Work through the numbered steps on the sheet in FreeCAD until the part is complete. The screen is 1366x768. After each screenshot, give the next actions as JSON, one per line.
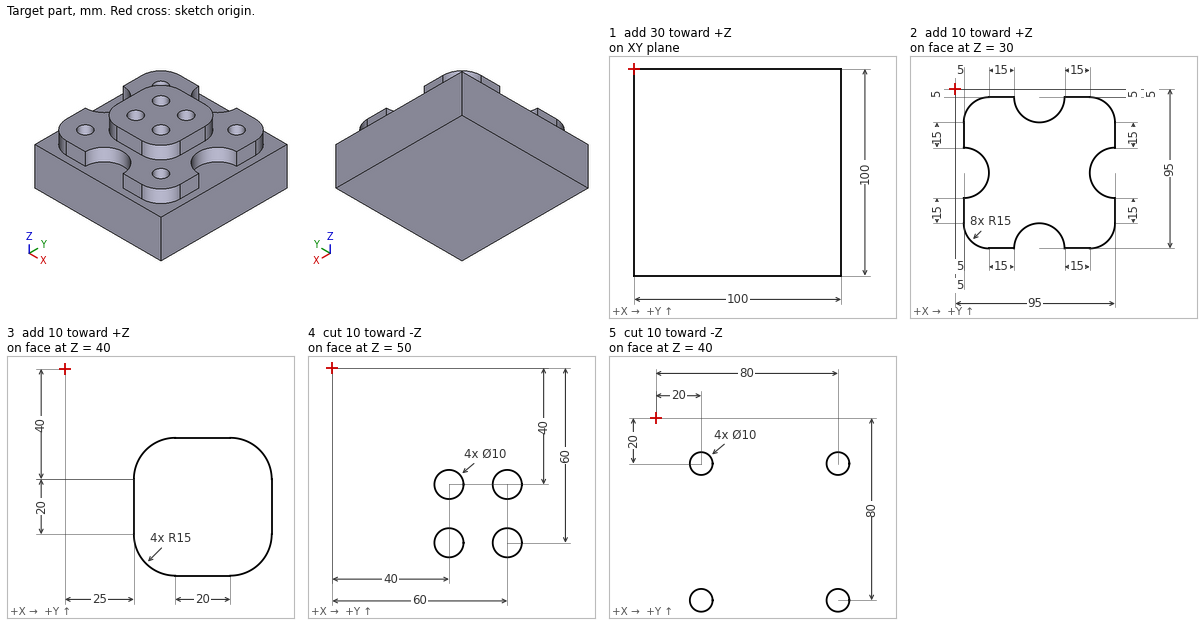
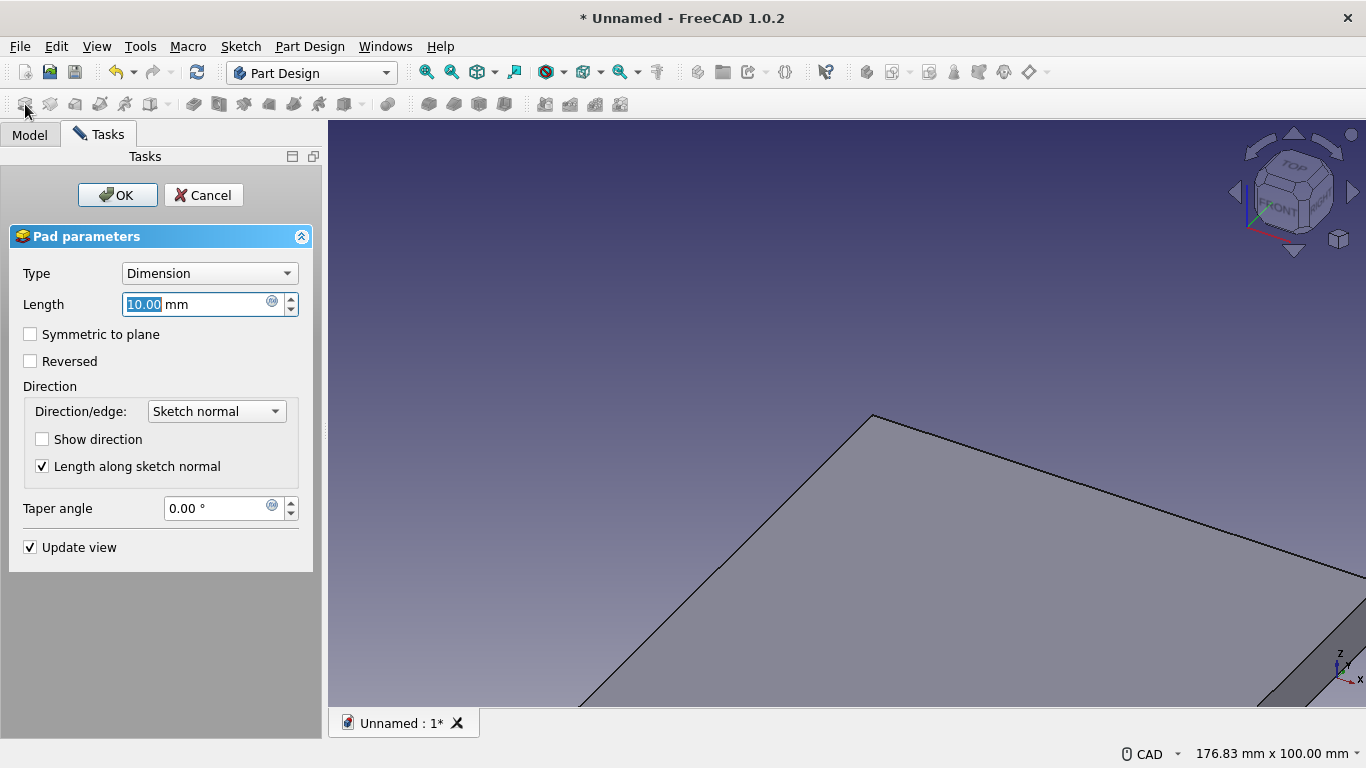
{"action": "type", "text": "30"}
{"action": "key", "text": "Tab"}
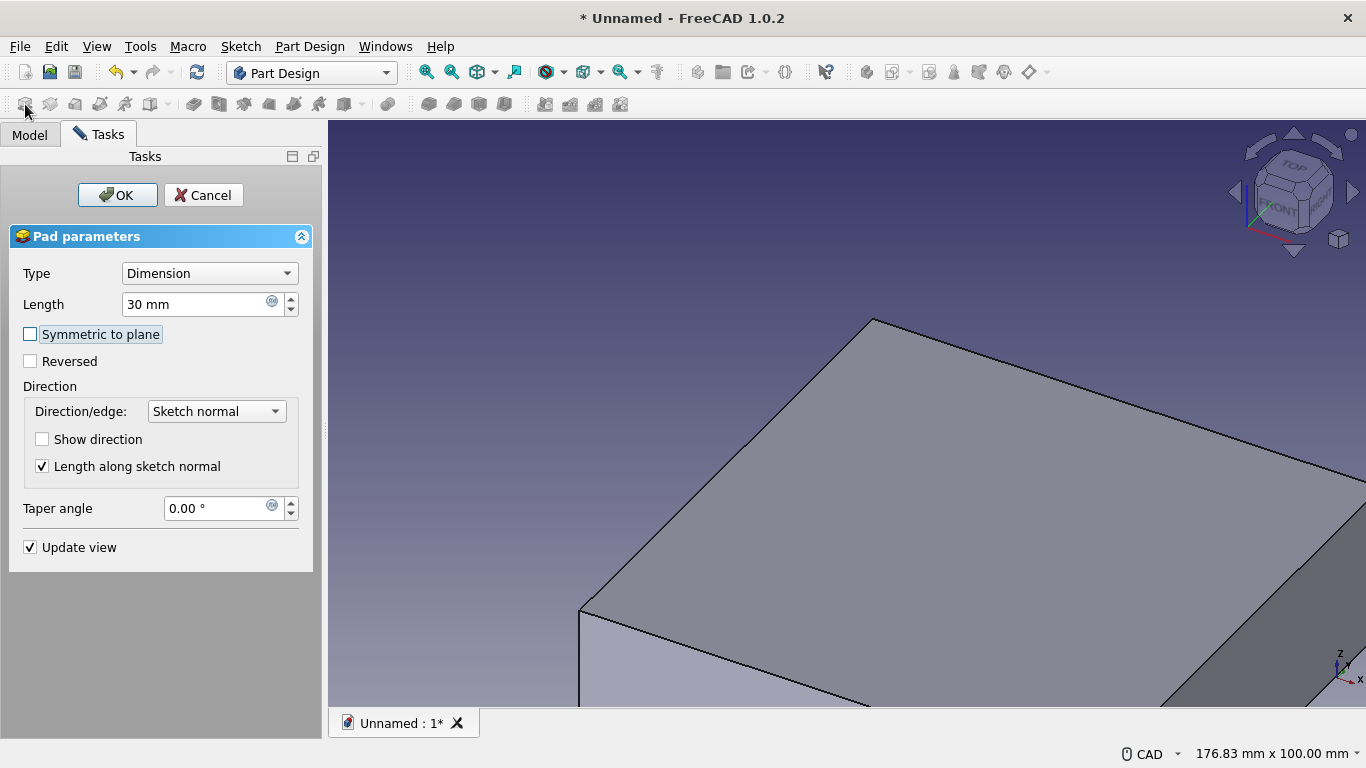
{"action": "left_click", "coordinate": [118, 195]}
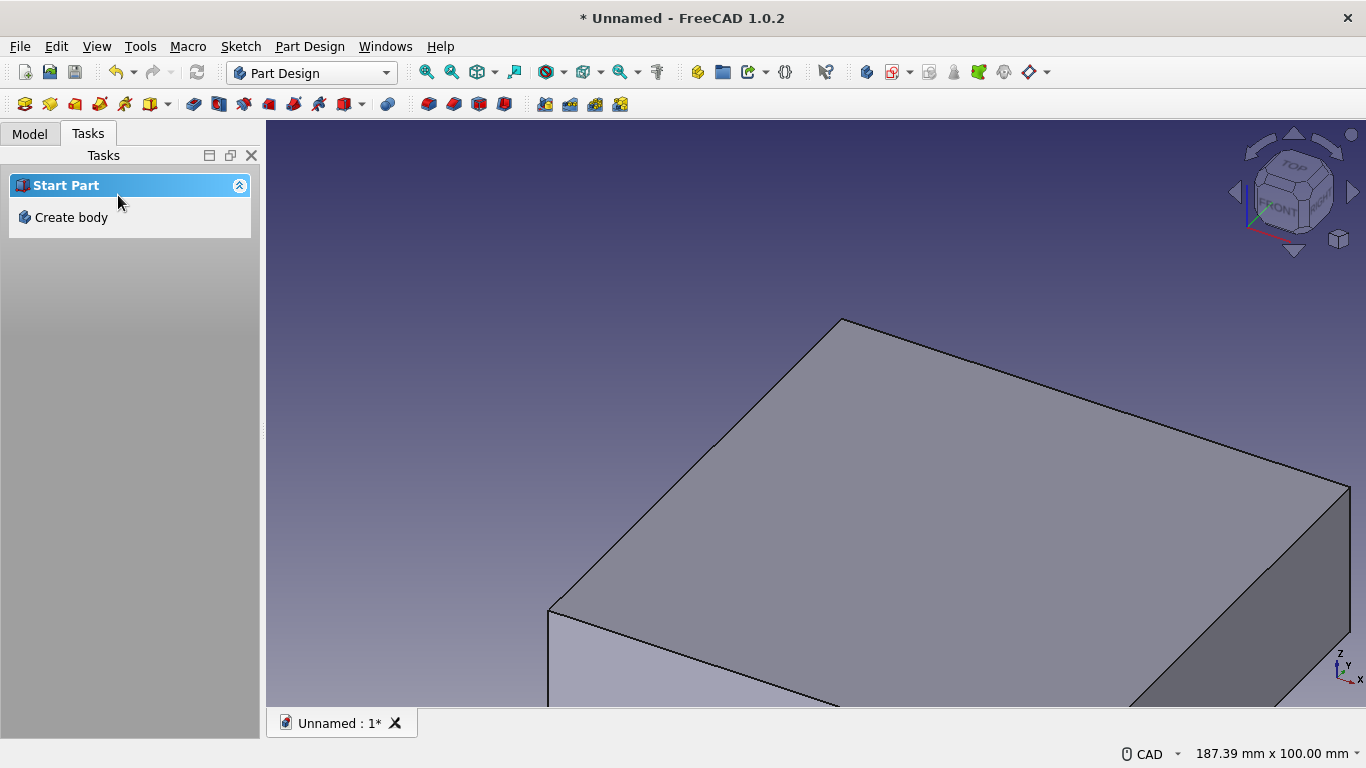
{"action": "left_click", "coordinate": [427, 72]}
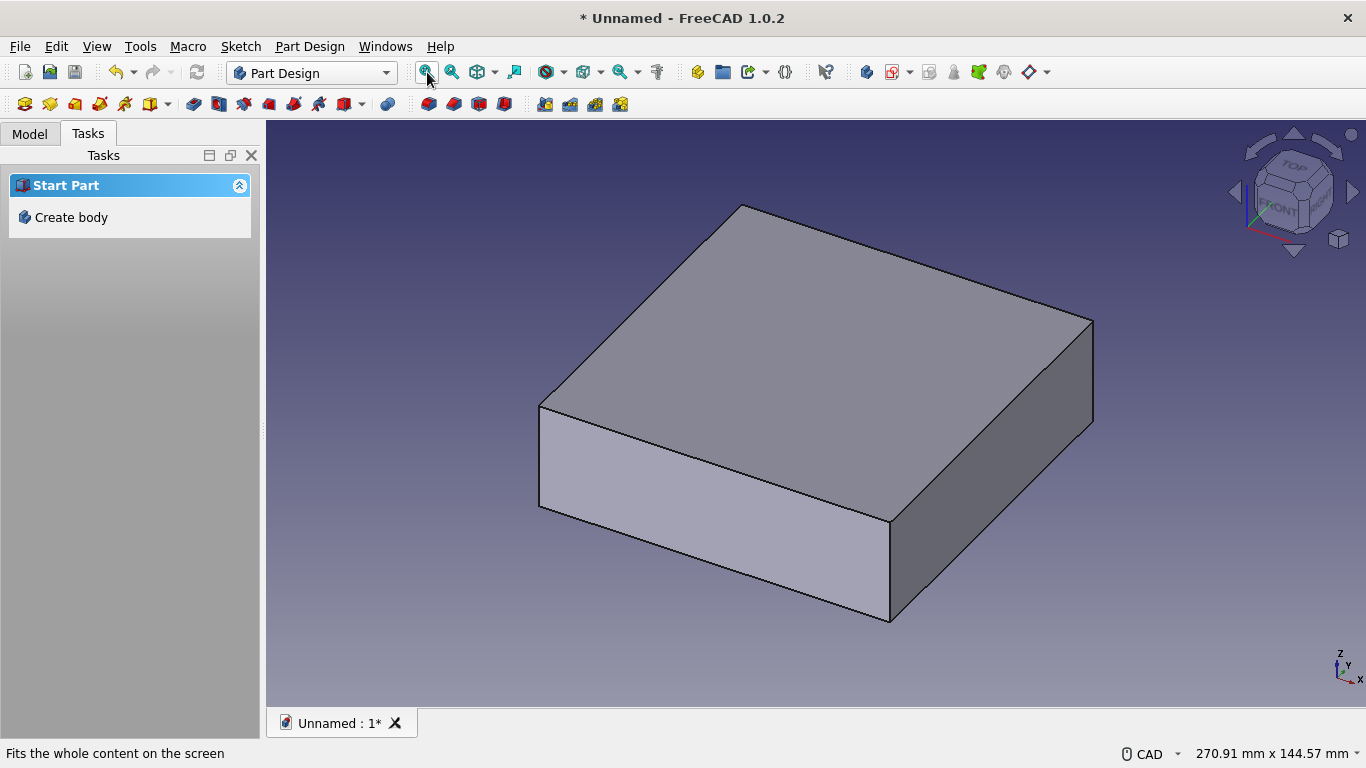
{"action": "left_click", "coordinate": [816, 363]}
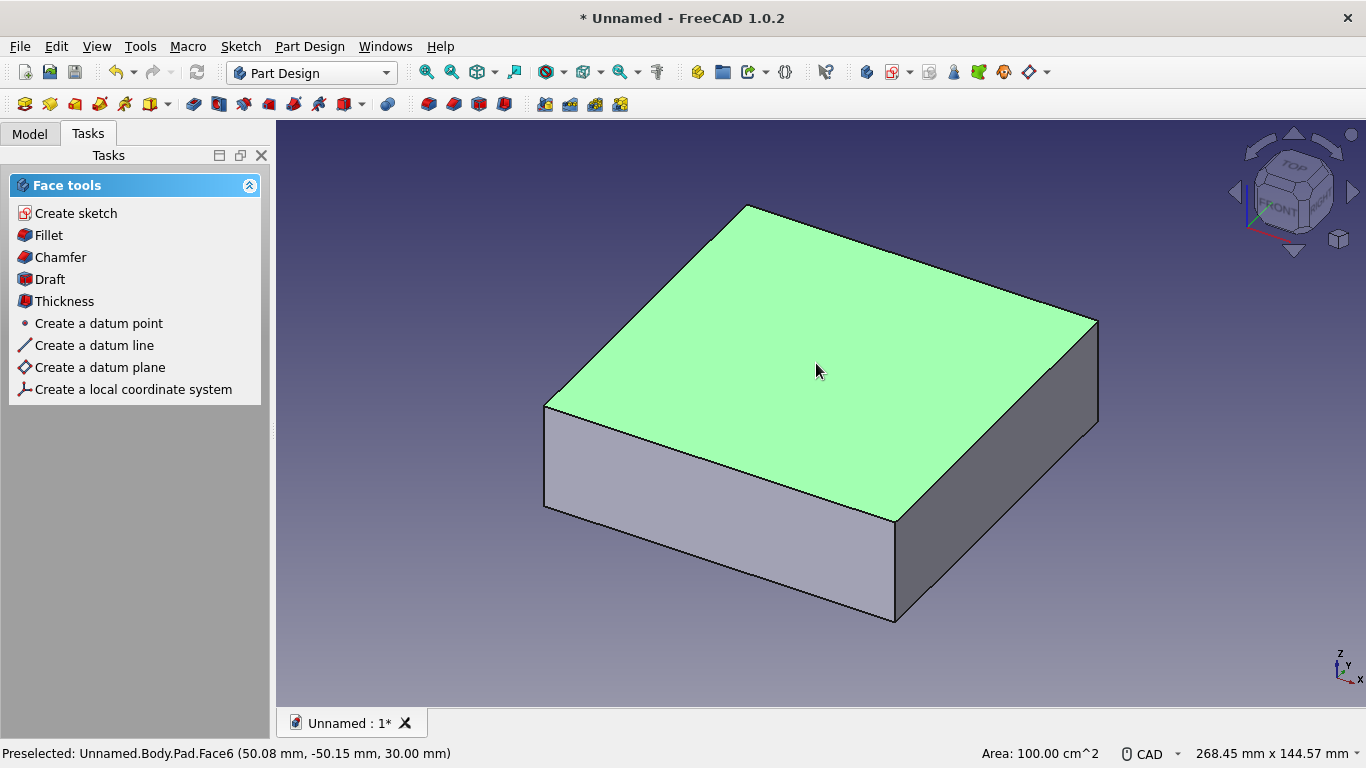
{"action": "left_click", "coordinate": [892, 72]}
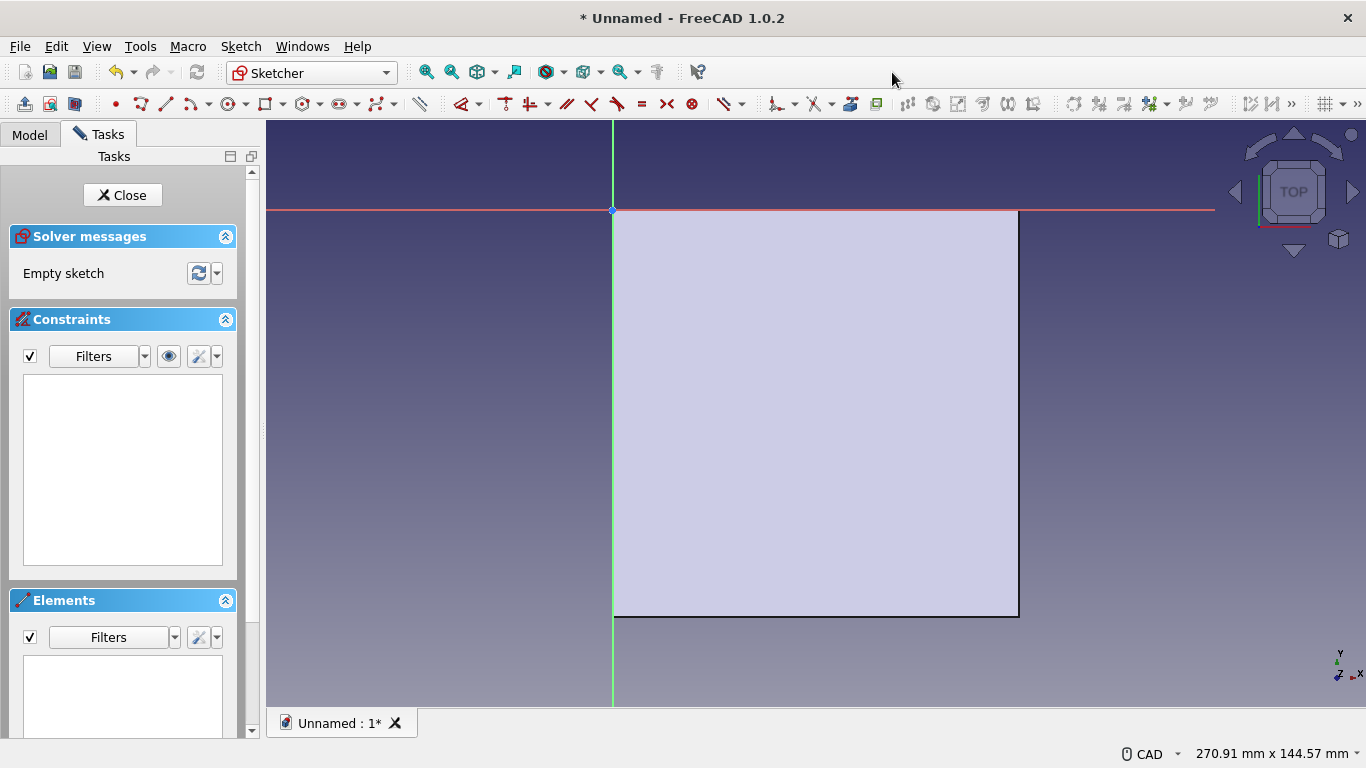
{"action": "left_click", "coordinate": [166, 104]}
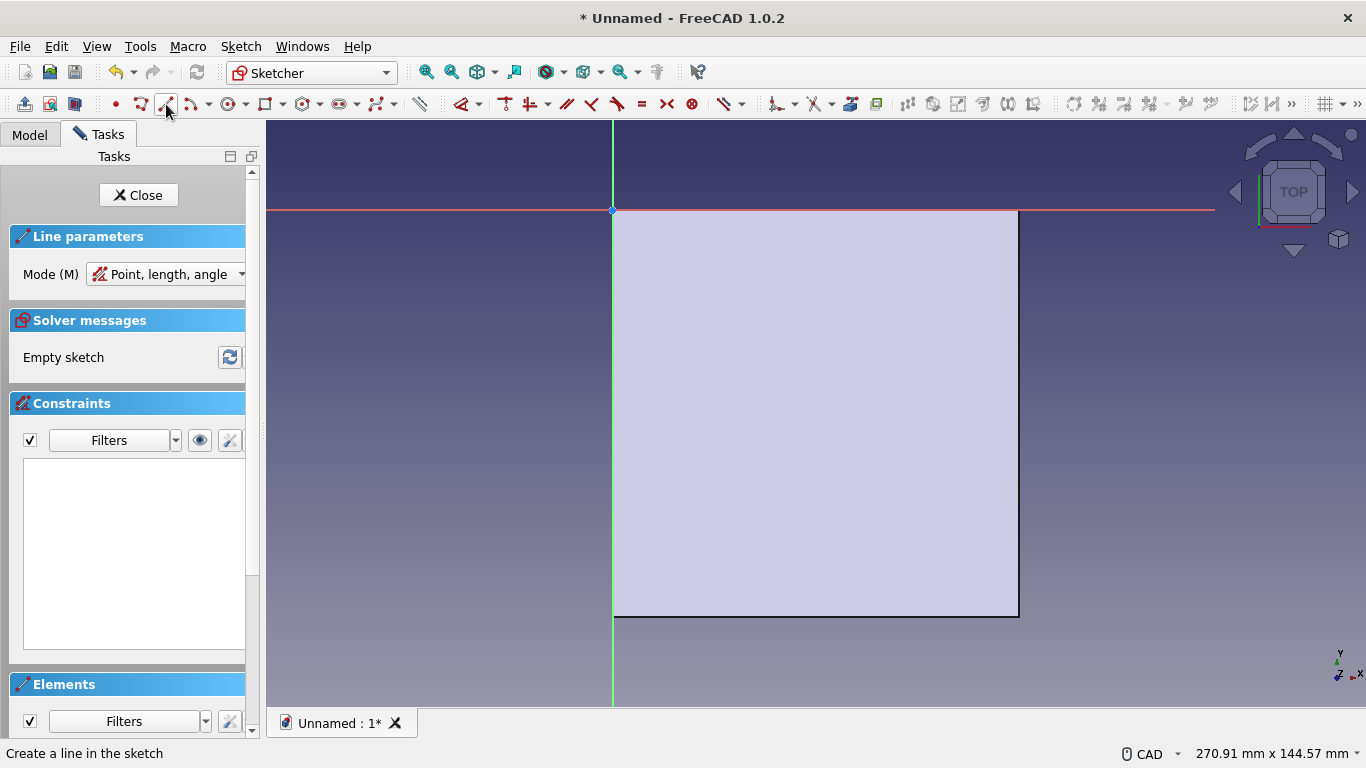
{"action": "left_click", "coordinate": [633, 474]}
{"action": "left_click", "coordinate": [633, 535]}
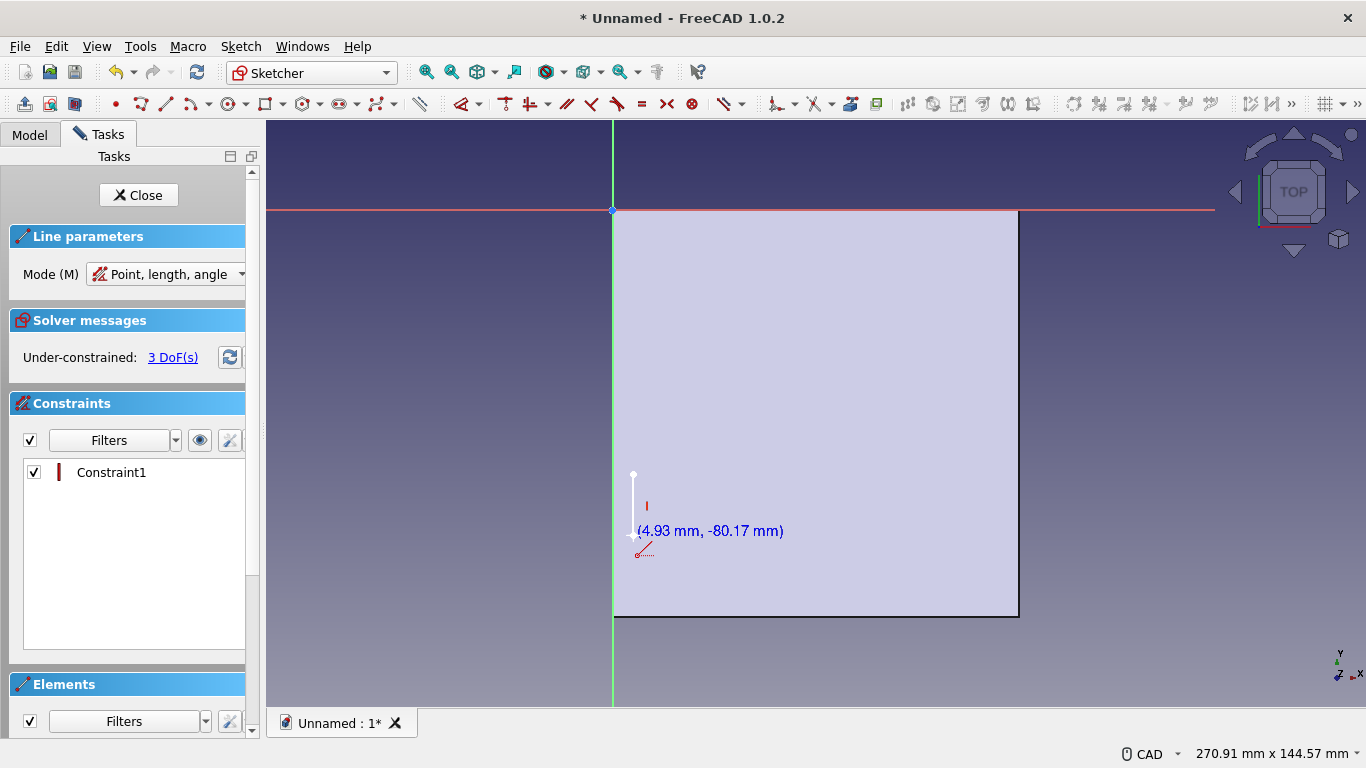
{"action": "left_click", "coordinate": [694, 596]}
{"action": "left_click", "coordinate": [755, 596]}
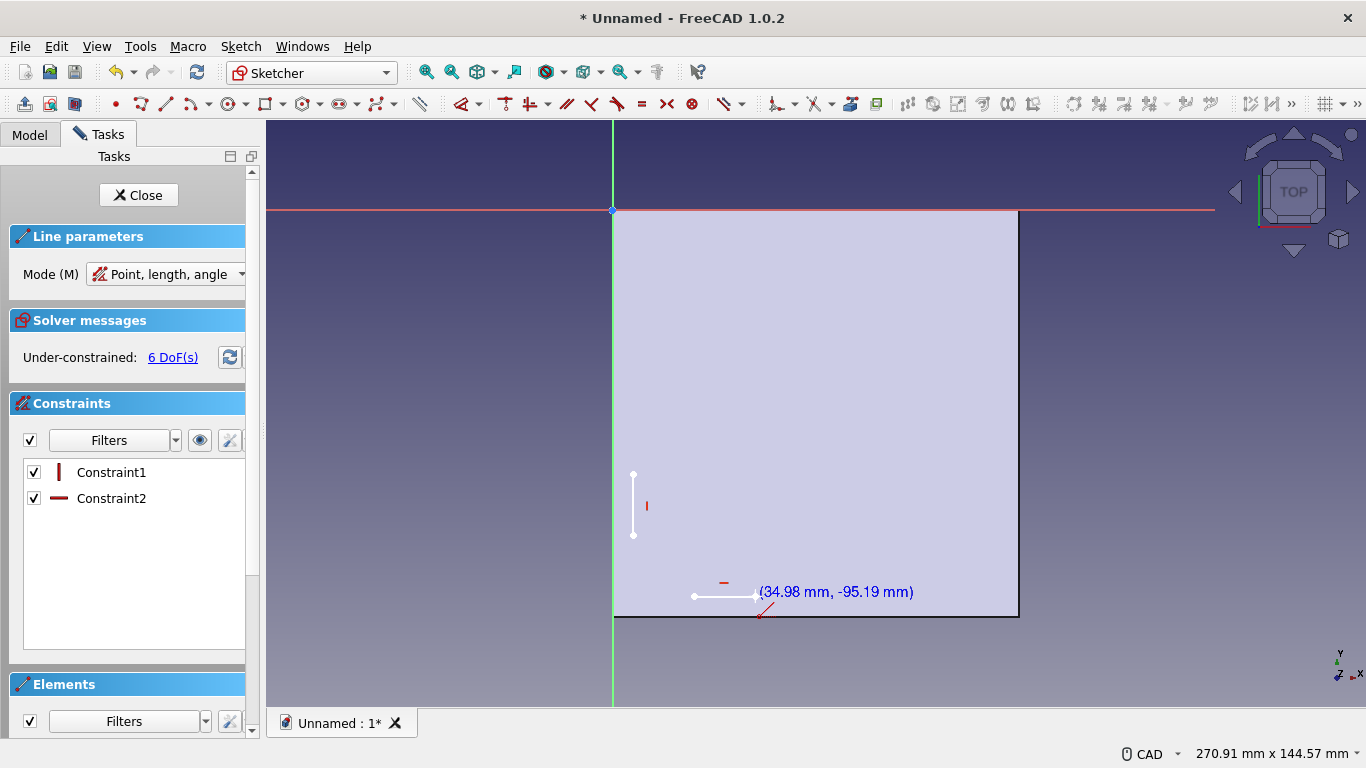
{"action": "left_click", "coordinate": [877, 596]}
{"action": "left_click", "coordinate": [938, 596]}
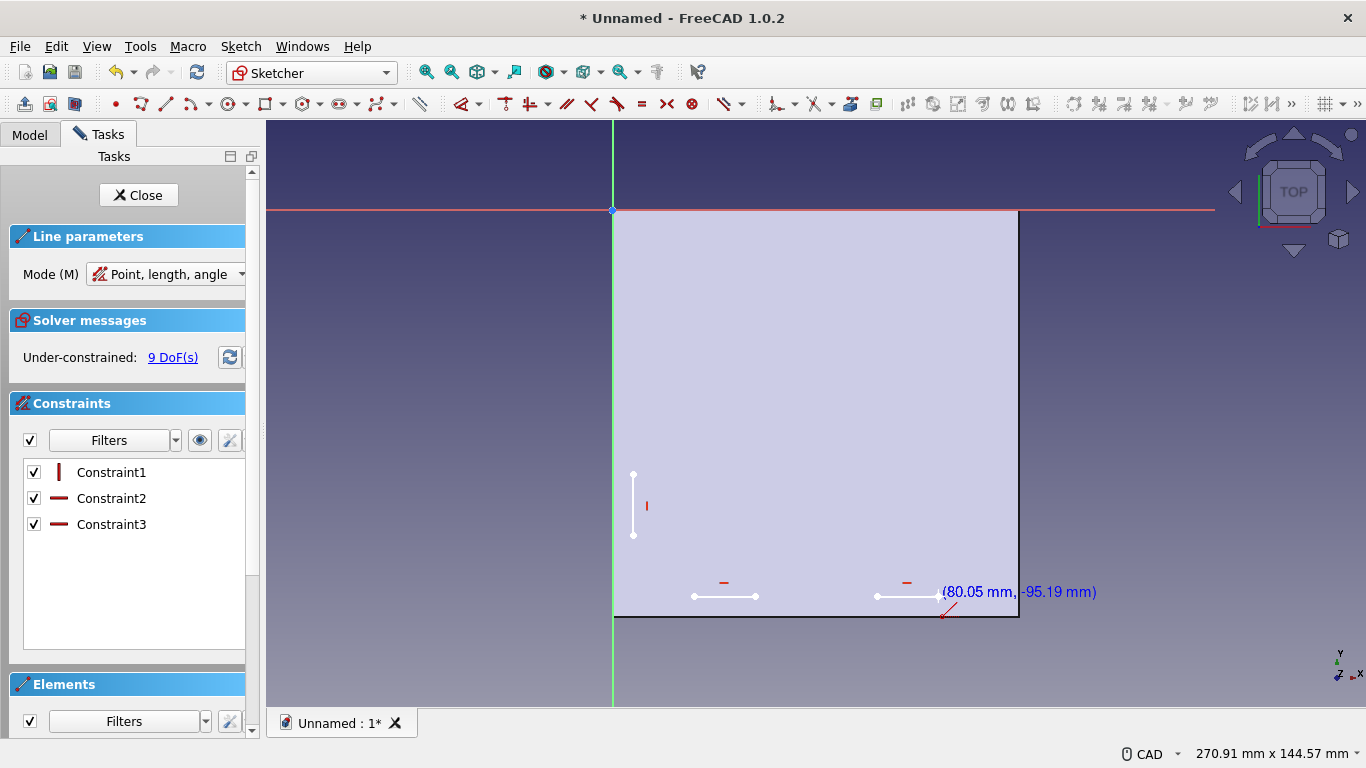
{"action": "left_click", "coordinate": [999, 535]}
{"action": "left_click", "coordinate": [999, 474]}